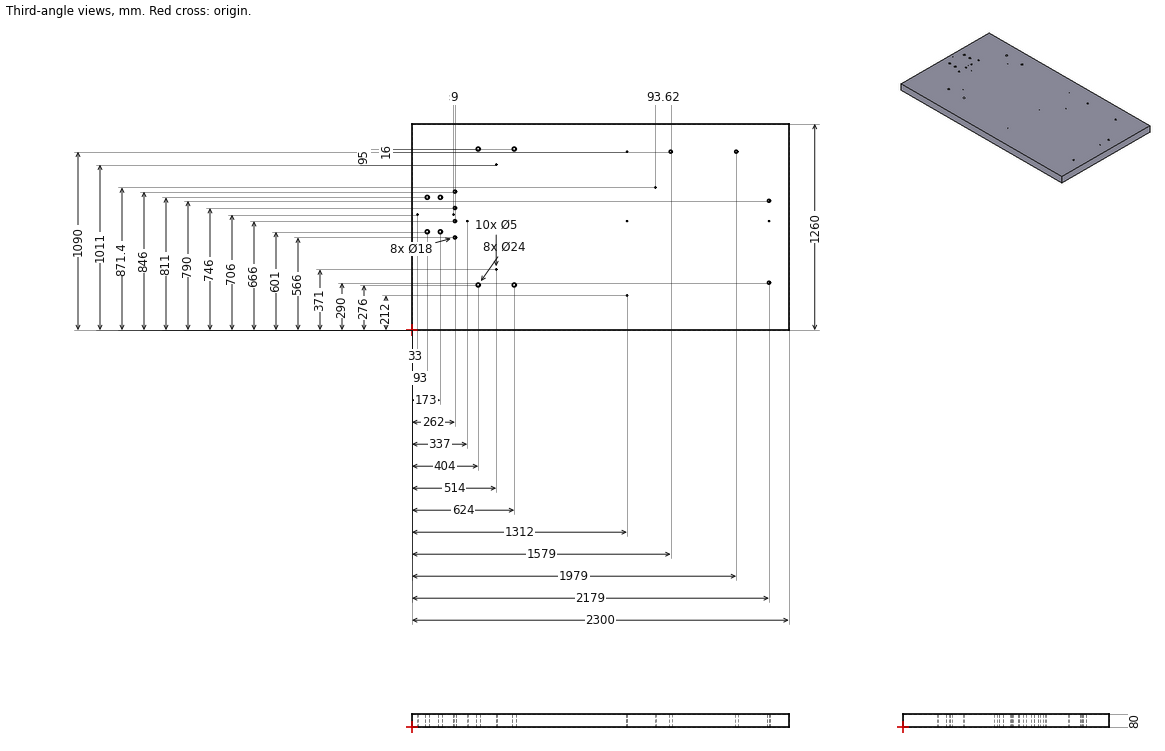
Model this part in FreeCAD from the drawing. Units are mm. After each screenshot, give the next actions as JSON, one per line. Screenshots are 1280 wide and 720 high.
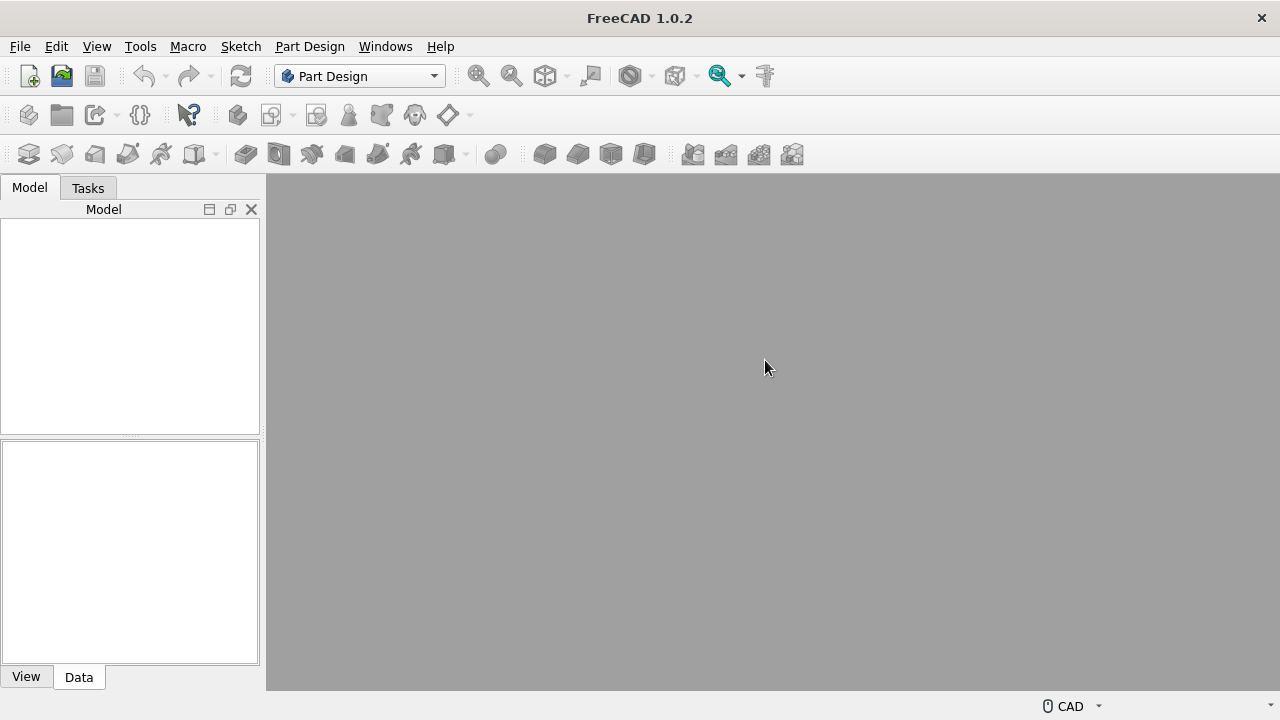
{"action": "left_click", "coordinate": [29, 76]}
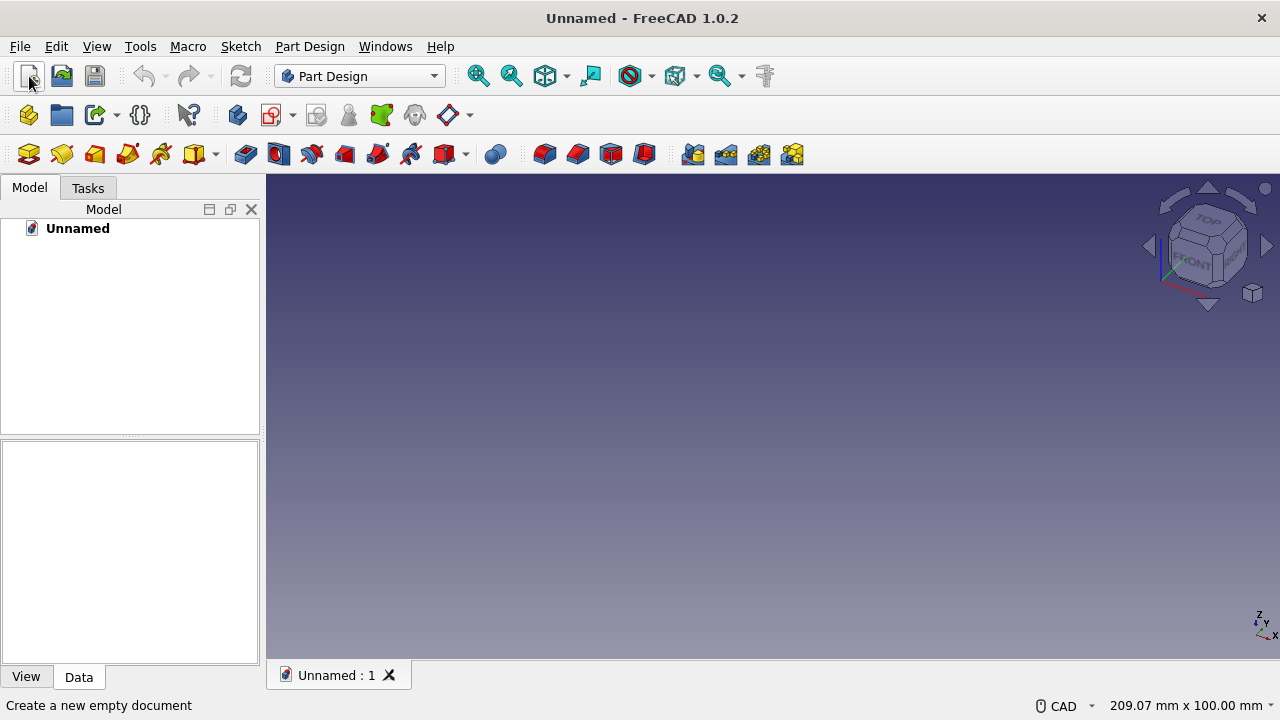
{"action": "left_click", "coordinate": [270, 116]}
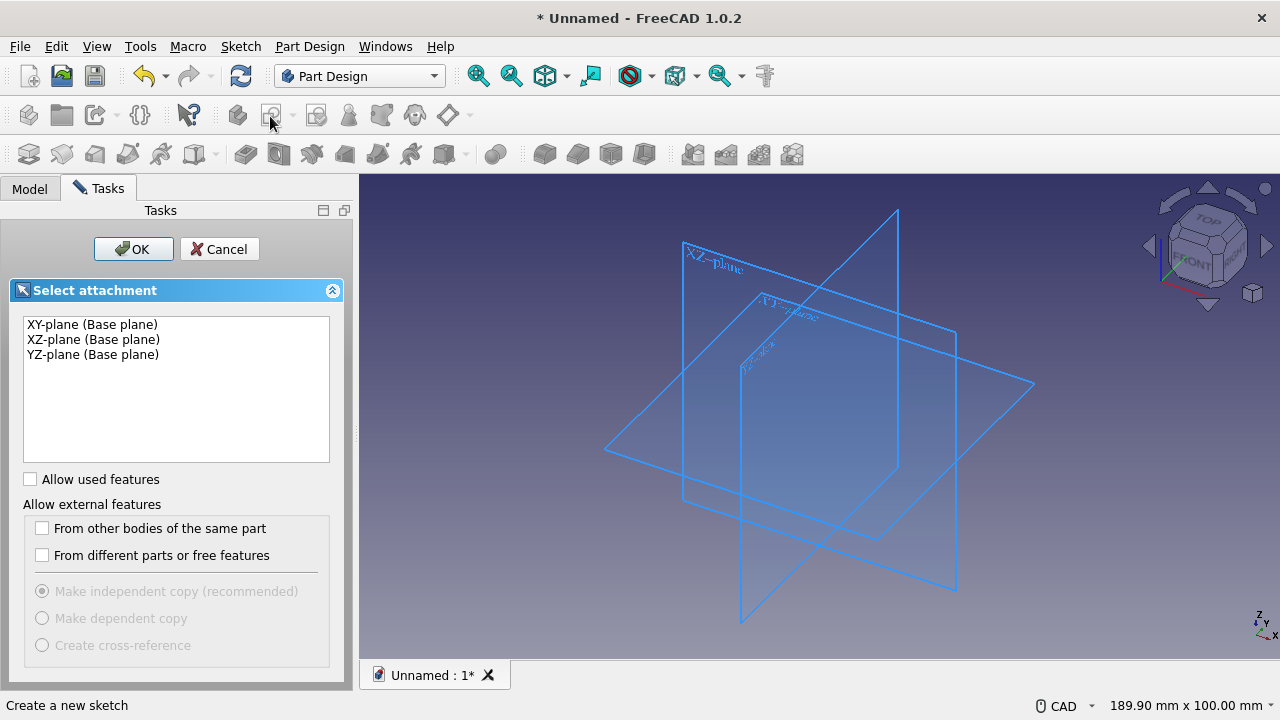
{"action": "left_click", "coordinate": [84, 324]}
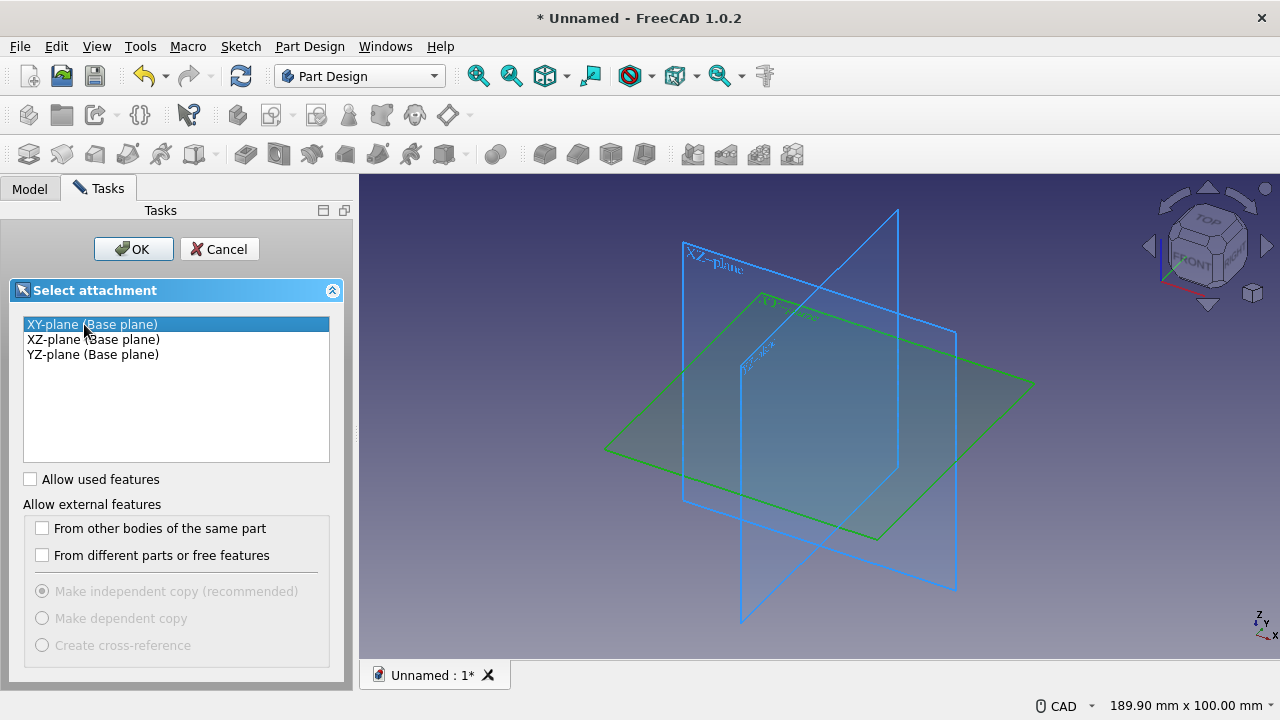
{"action": "left_click", "coordinate": [134, 249]}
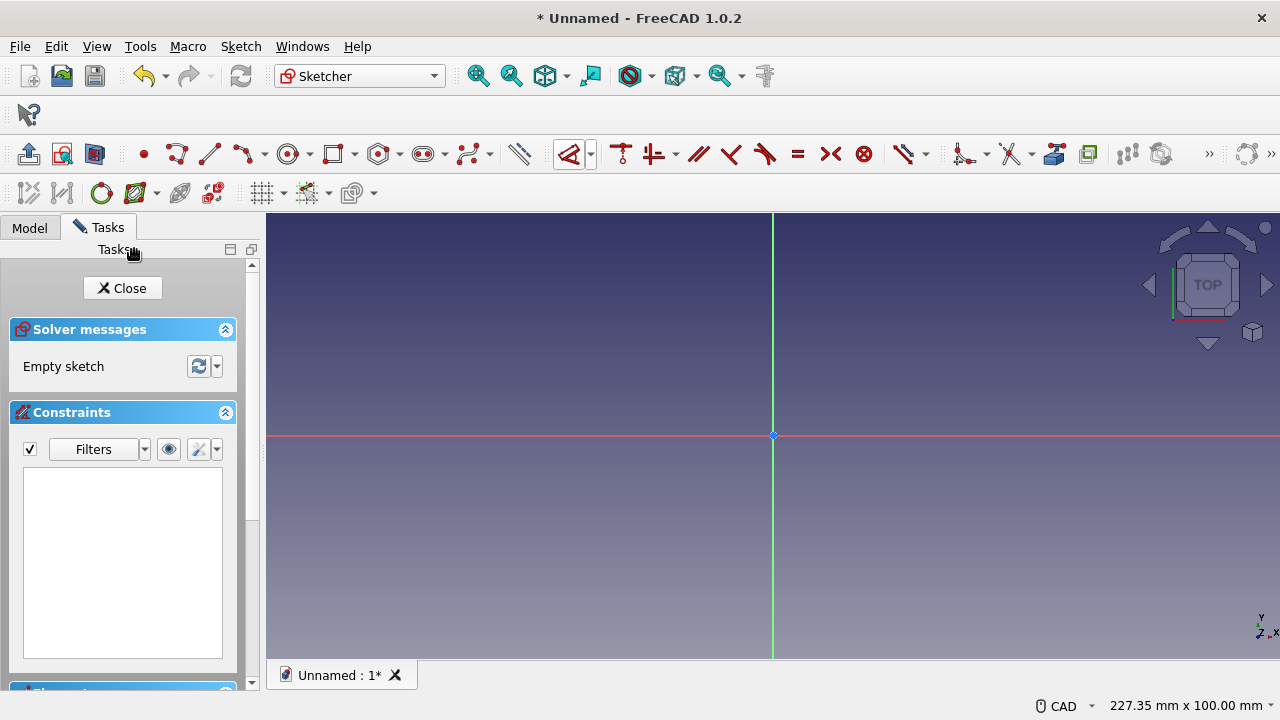
{"action": "scroll", "coordinate": [432, 583], "scroll_direction": "down", "scroll_amount": 15}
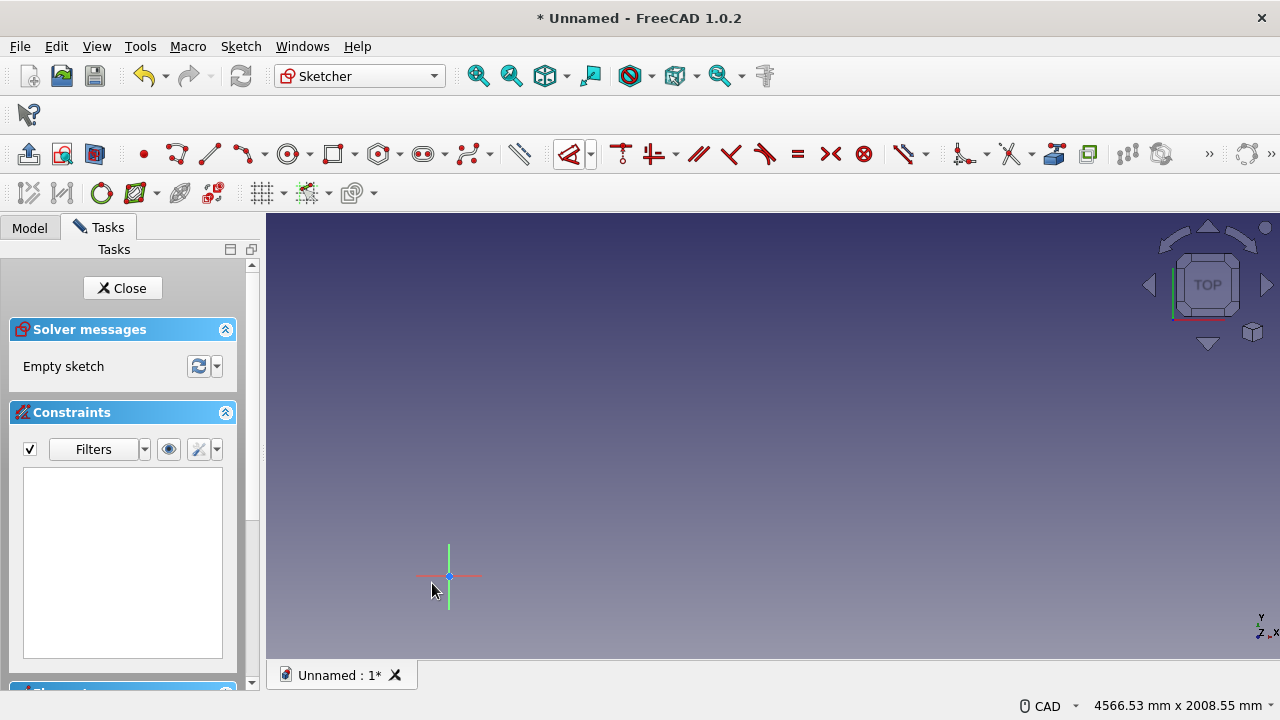
{"action": "left_click", "coordinate": [332, 154]}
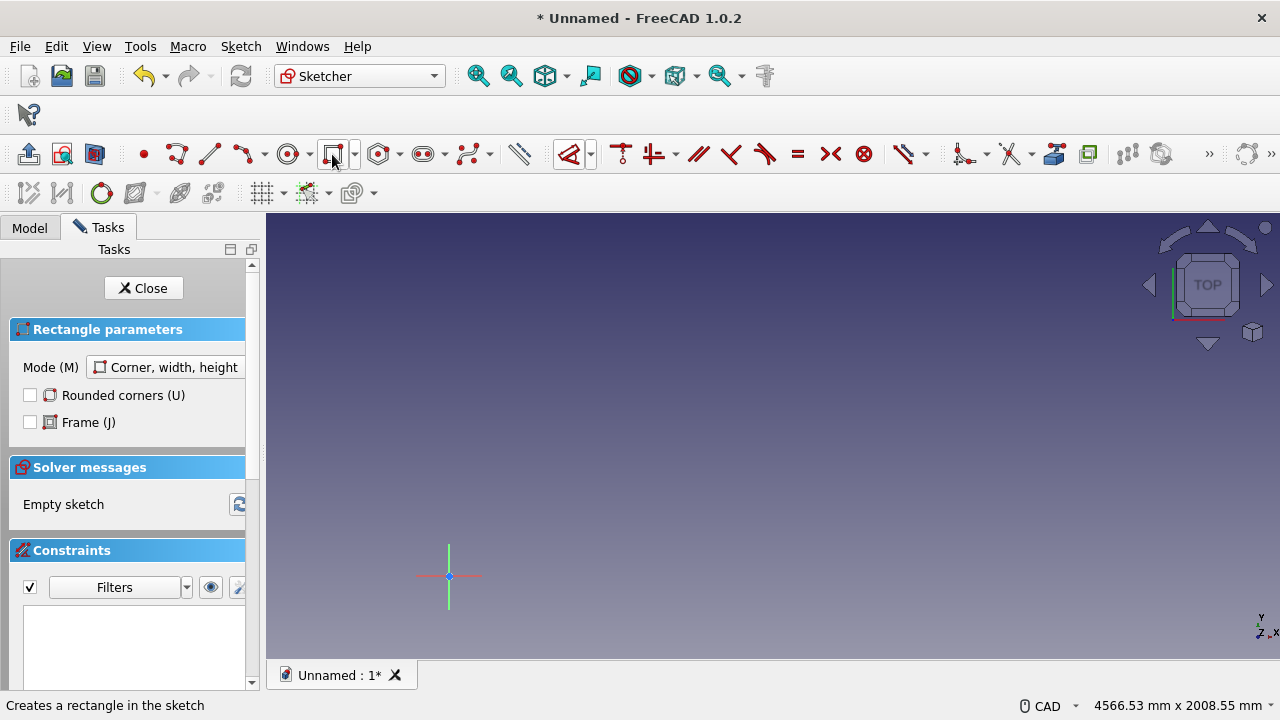
{"action": "left_click", "coordinate": [449, 576]}
{"action": "left_click", "coordinate": [960, 297]}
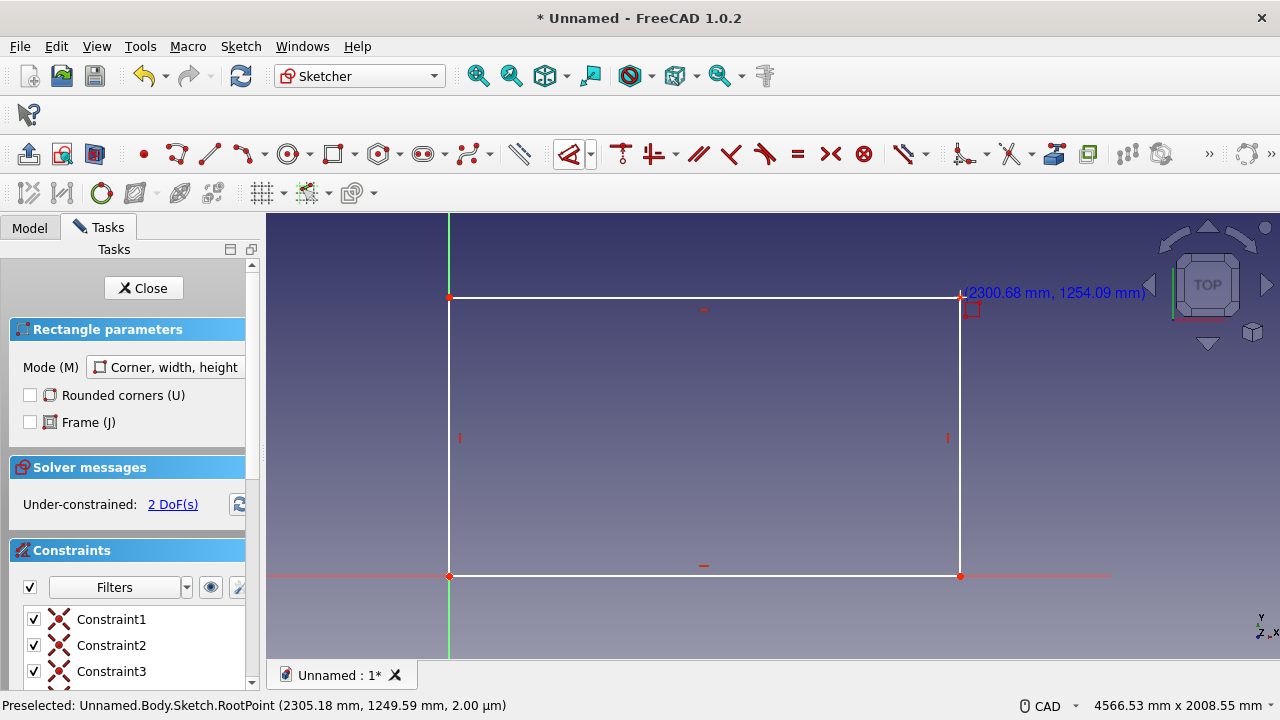
{"action": "left_click", "coordinate": [288, 154]}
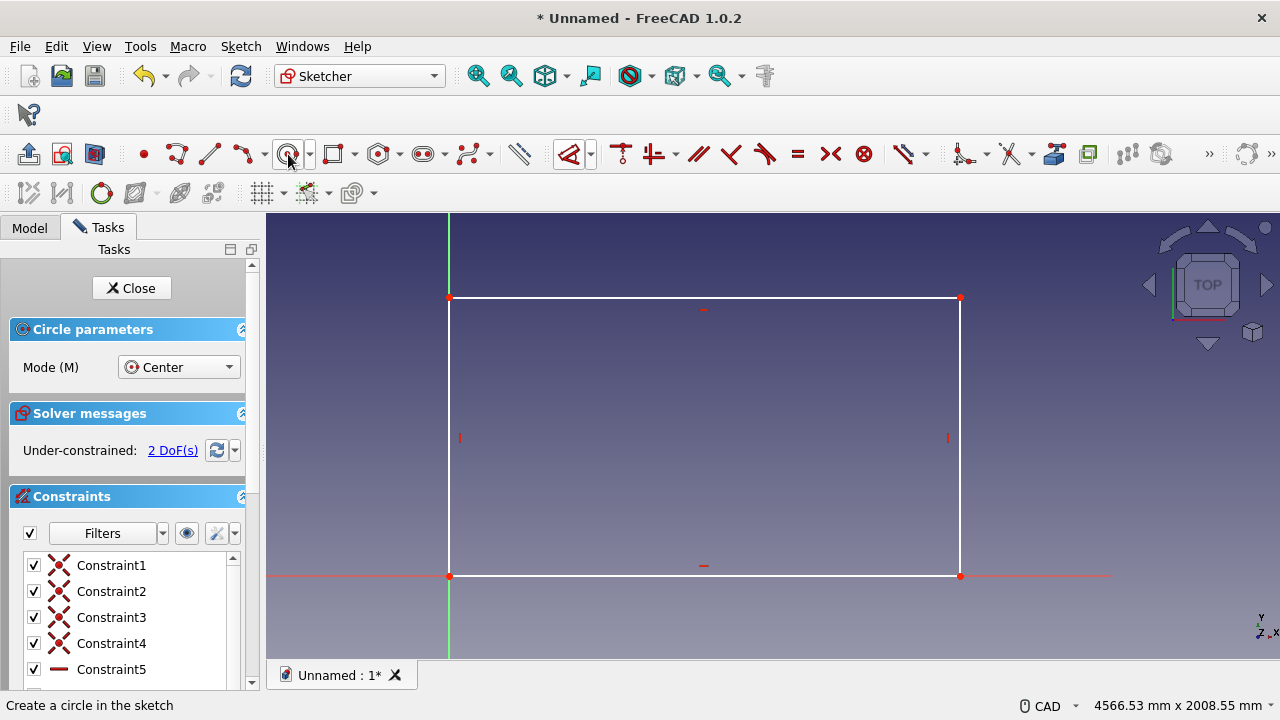
{"action": "scroll", "coordinate": [539, 515], "scroll_direction": "up", "scroll_amount": 11}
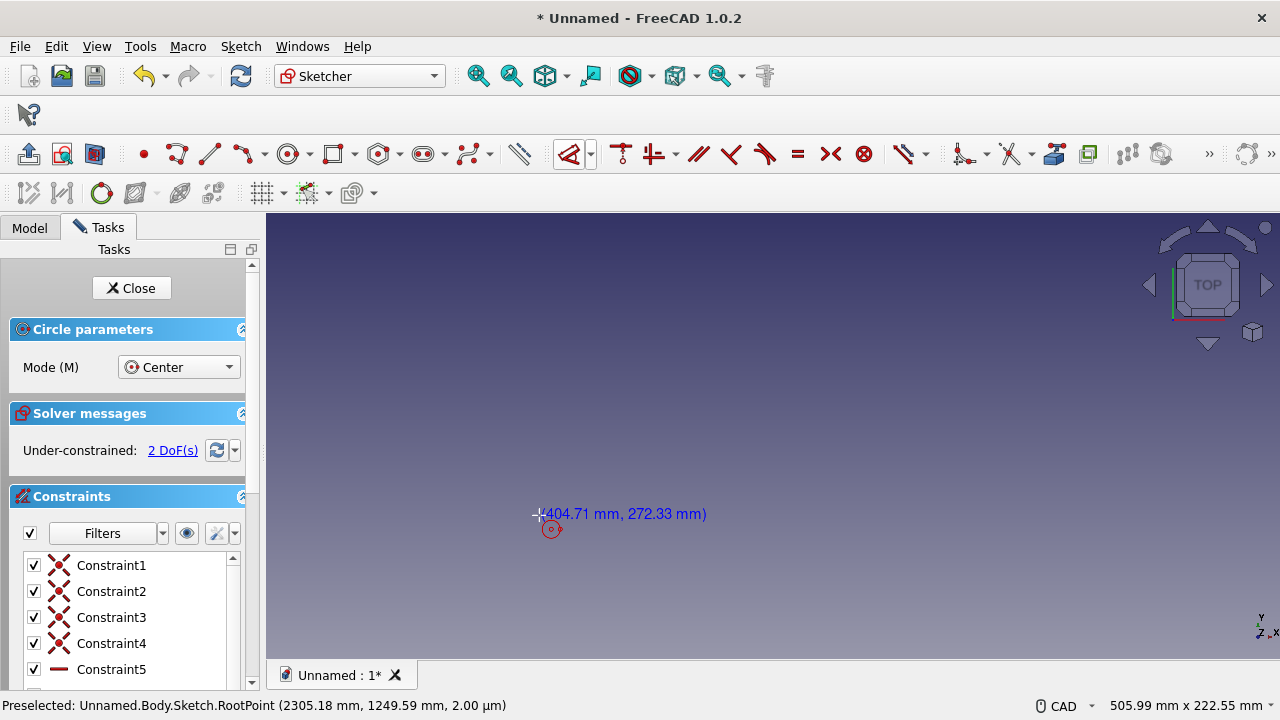
{"action": "scroll", "coordinate": [539, 515], "scroll_direction": "down", "scroll_amount": 11}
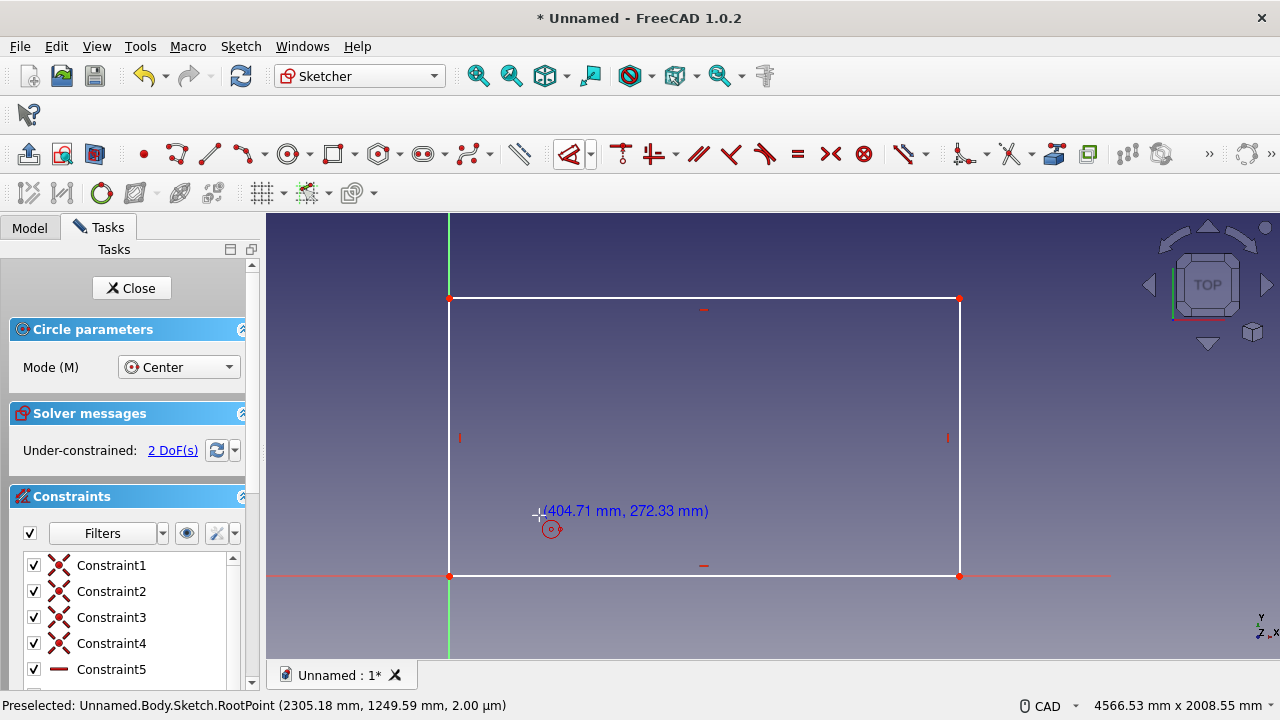
{"action": "left_click", "coordinate": [539, 515]}